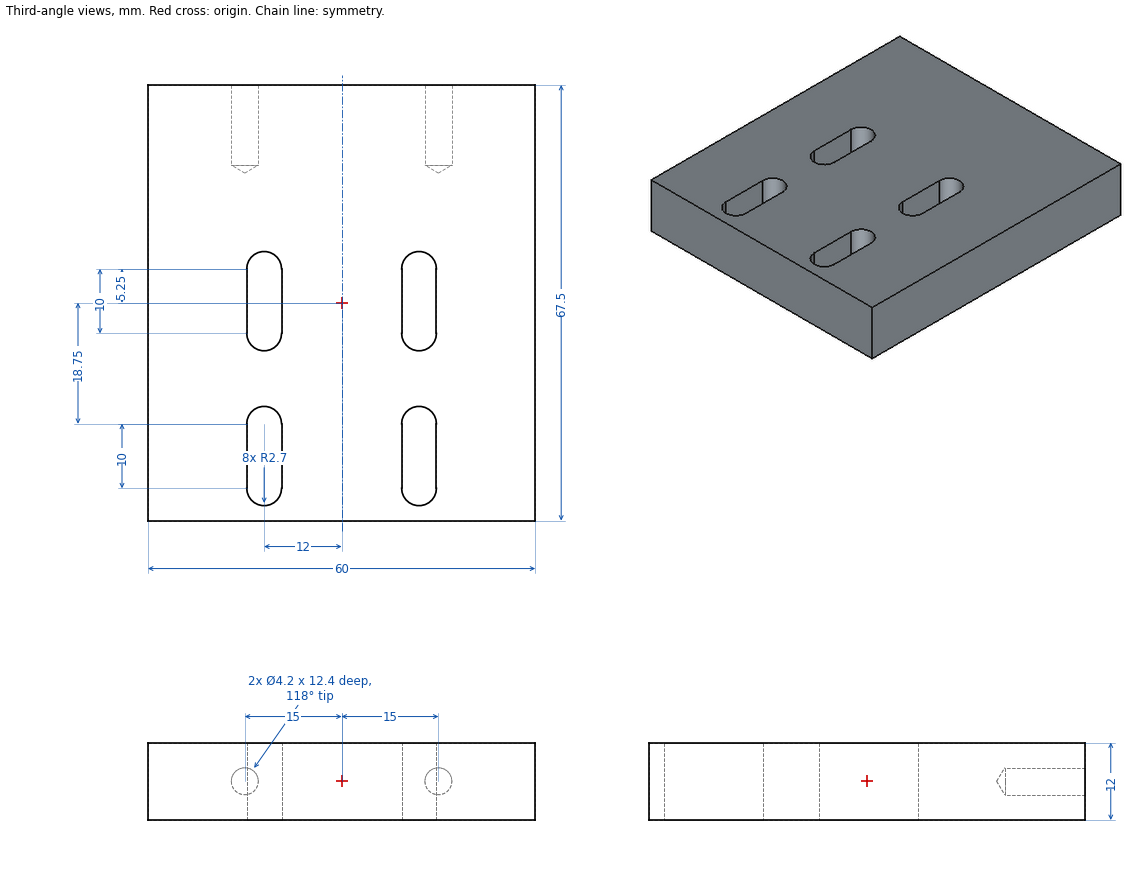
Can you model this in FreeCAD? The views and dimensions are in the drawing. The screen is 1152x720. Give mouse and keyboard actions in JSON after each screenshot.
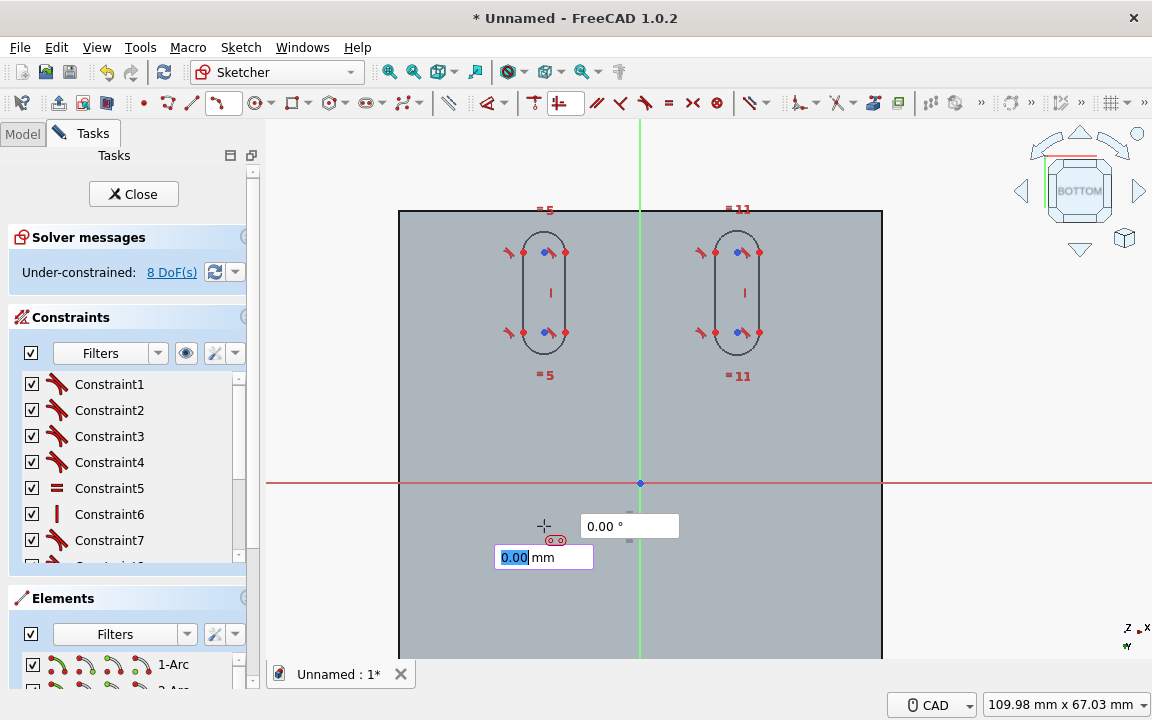
{"action": "left_click", "coordinate": [544, 445]}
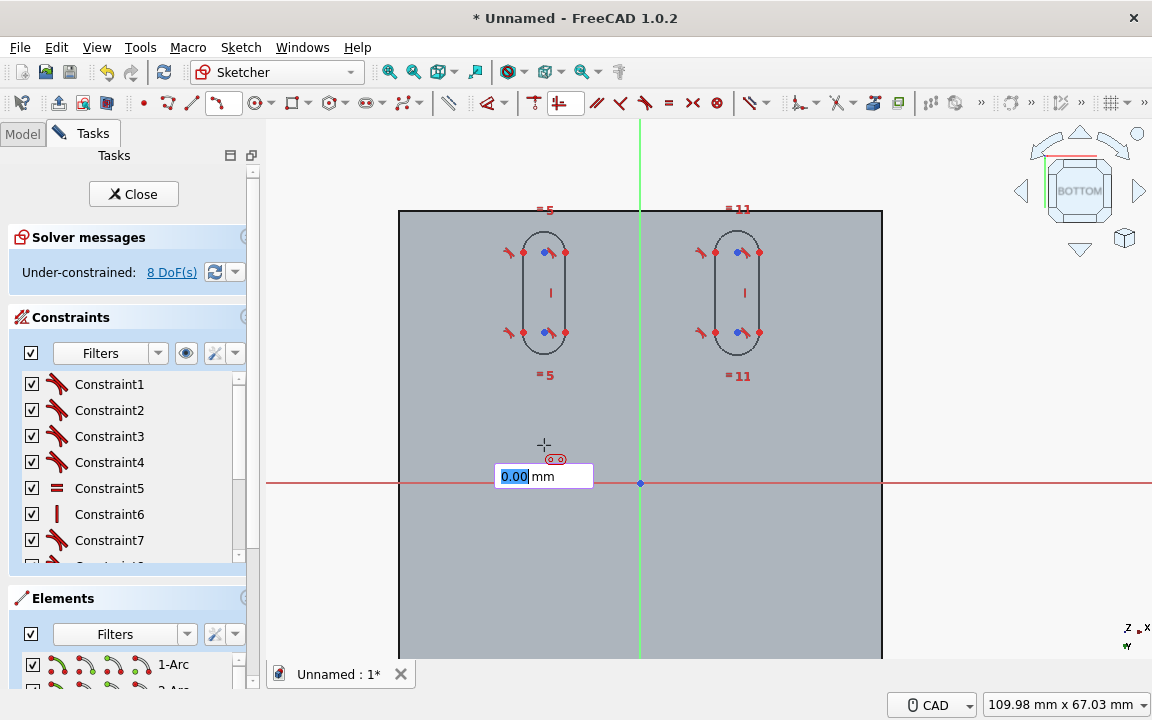
{"action": "left_click", "coordinate": [522, 497]}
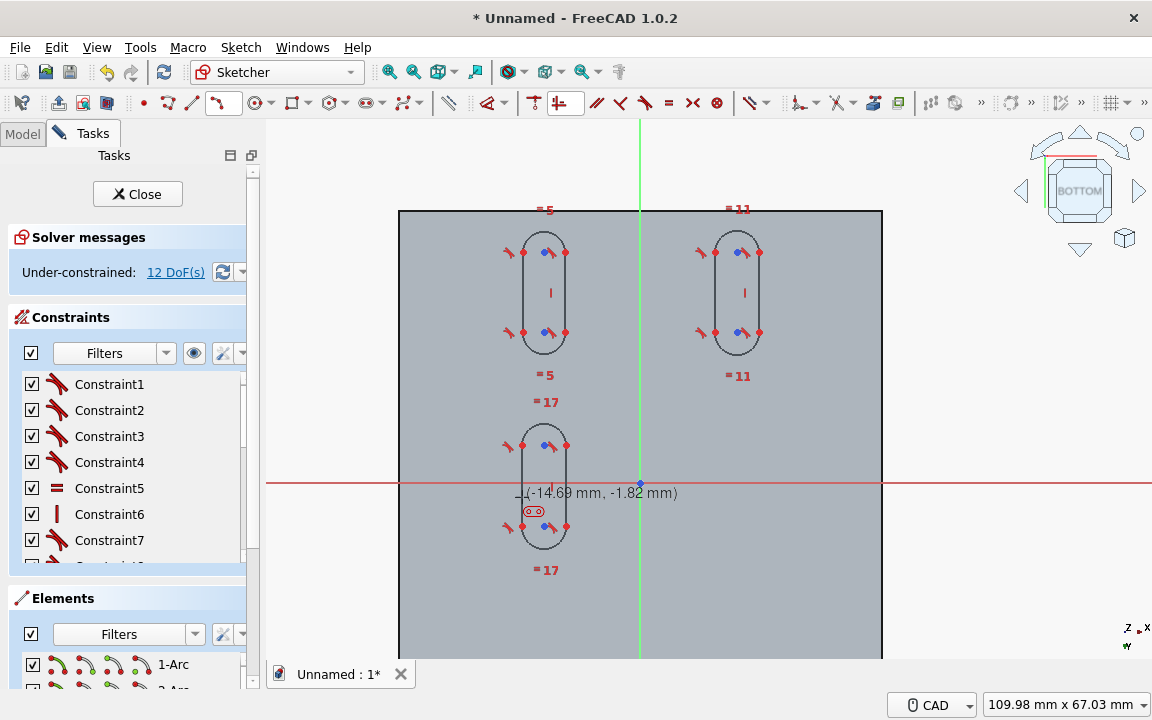
{"action": "left_click", "coordinate": [737, 526]}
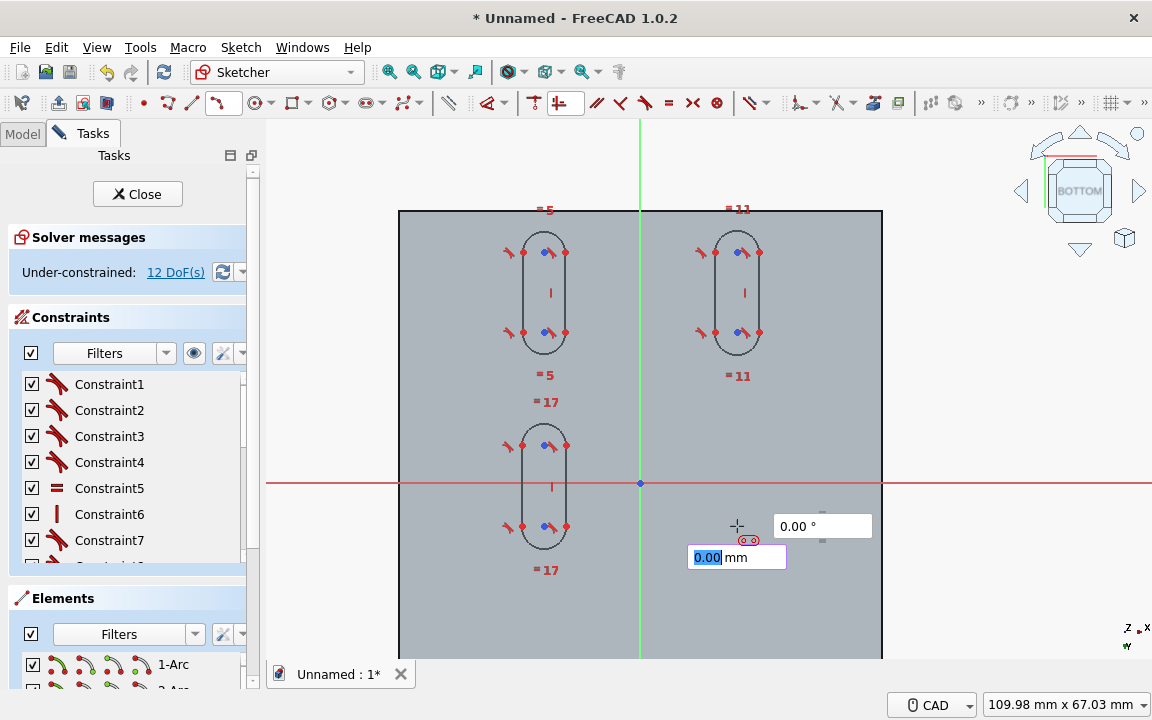
{"action": "left_click", "coordinate": [737, 445]}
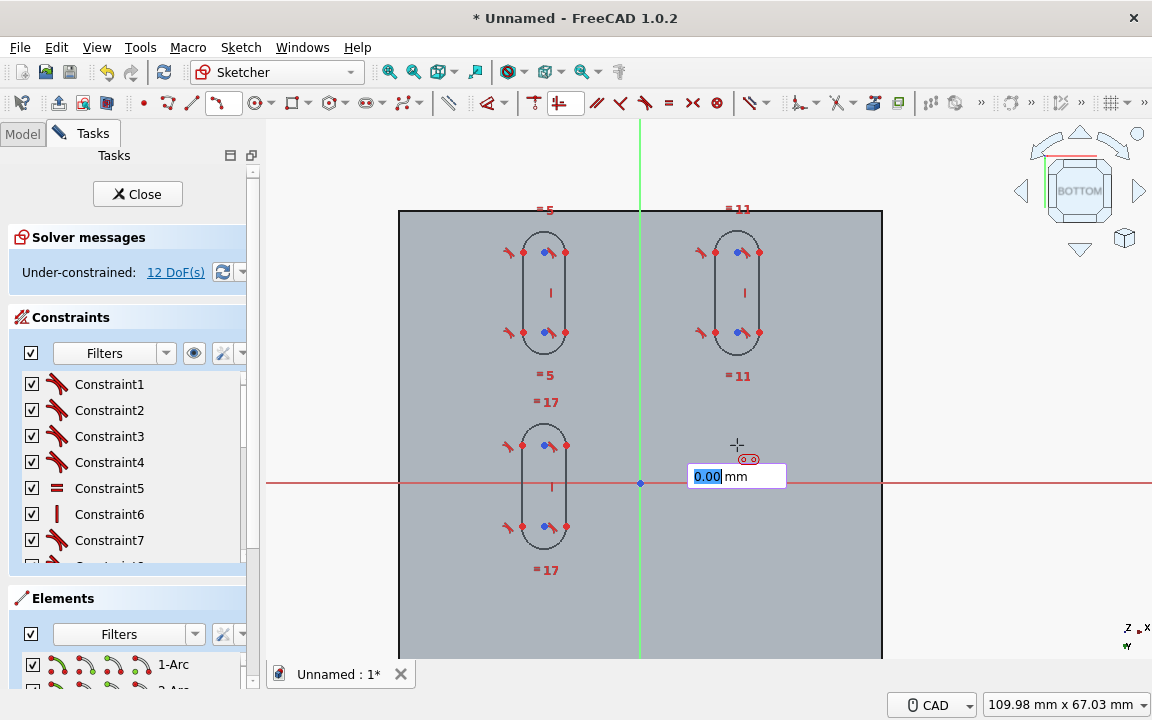
{"action": "left_click", "coordinate": [715, 497]}
{"action": "key", "text": "Escape"}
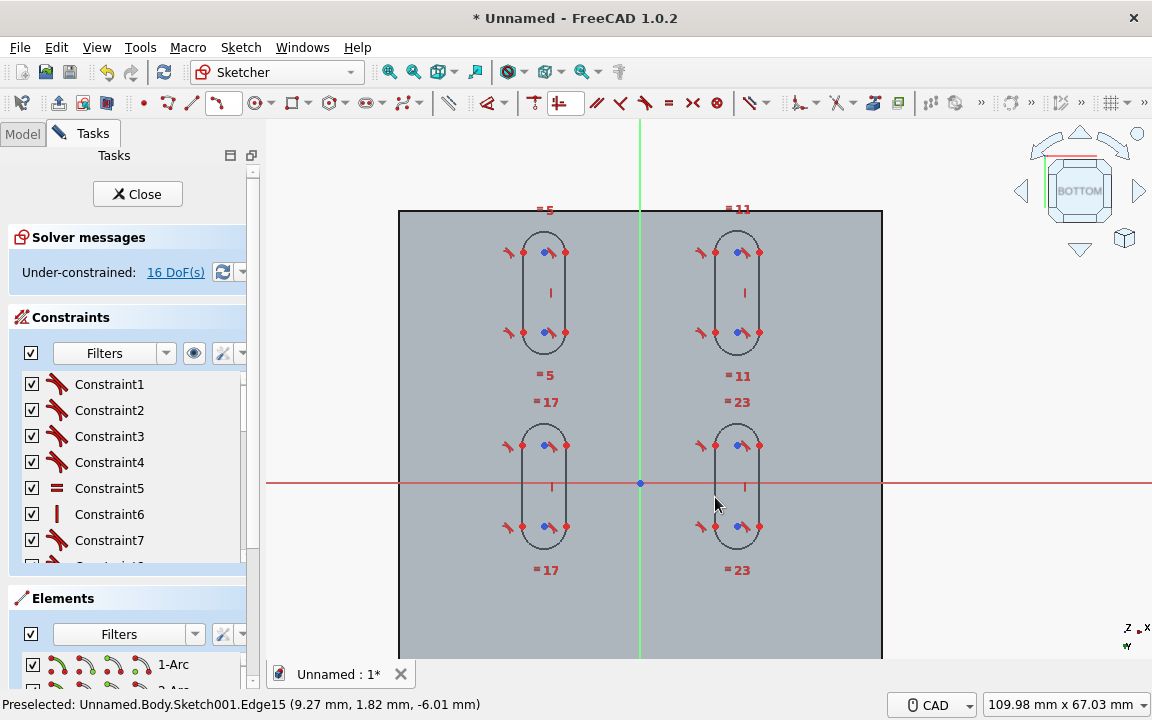
{"action": "left_click", "coordinate": [532, 350]}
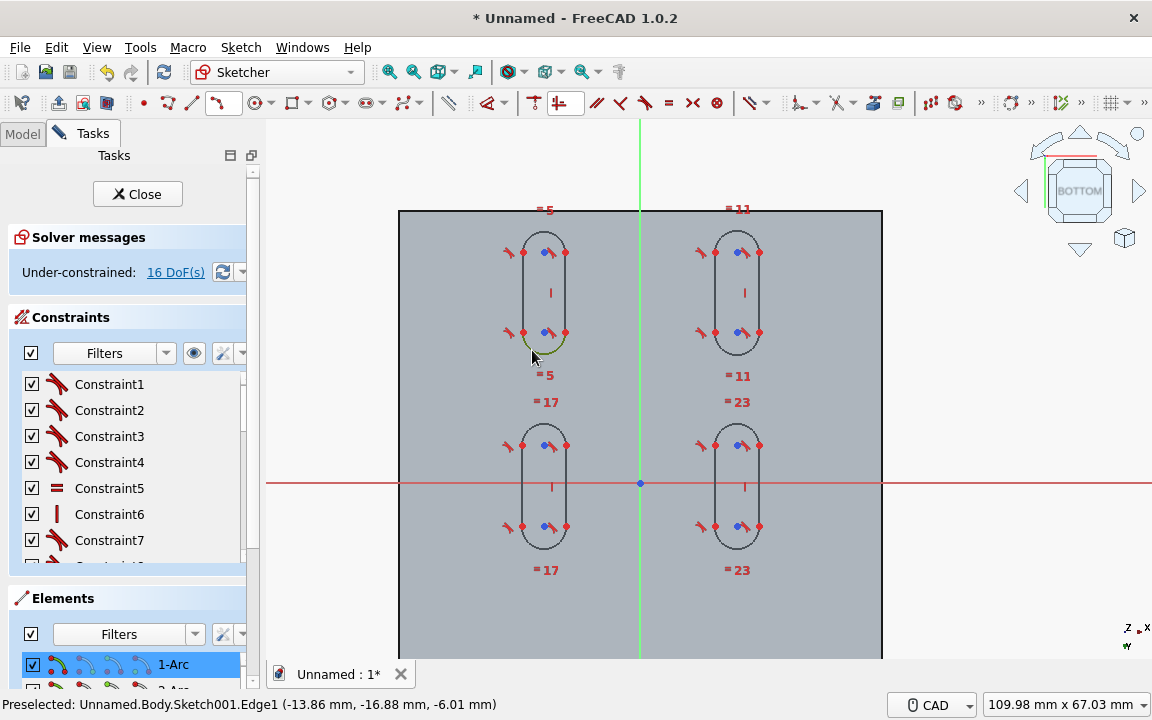
{"action": "left_click", "coordinate": [724, 351]}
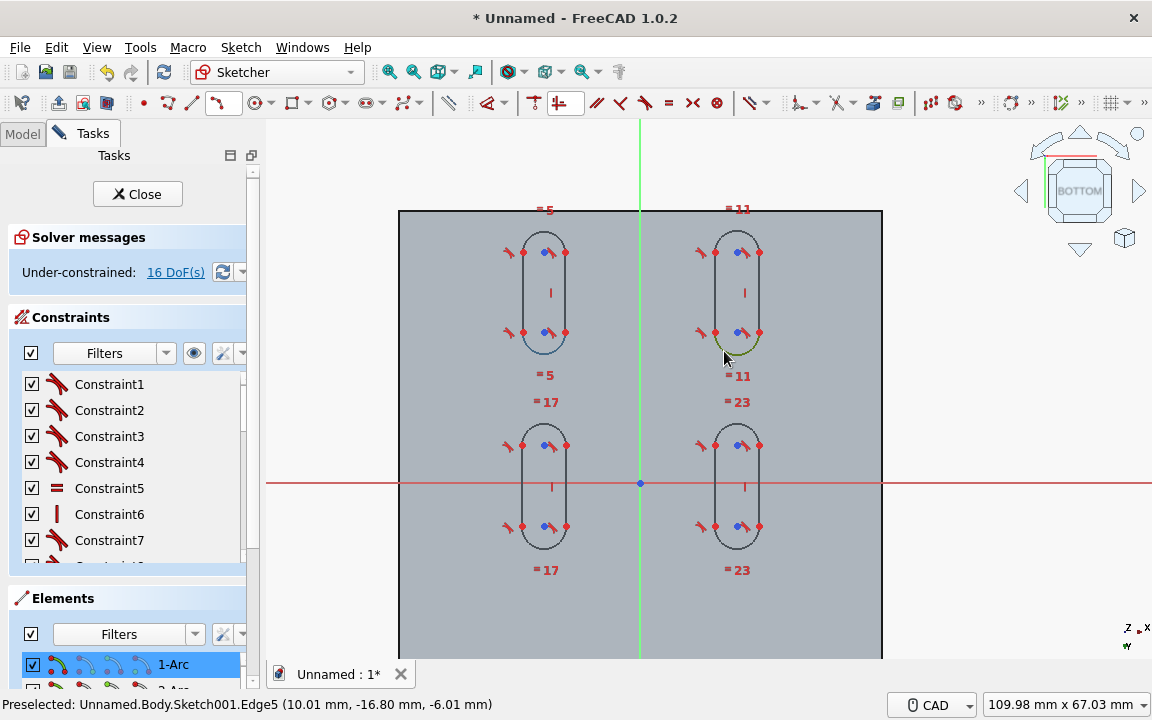
{"action": "left_click", "coordinate": [531, 545]}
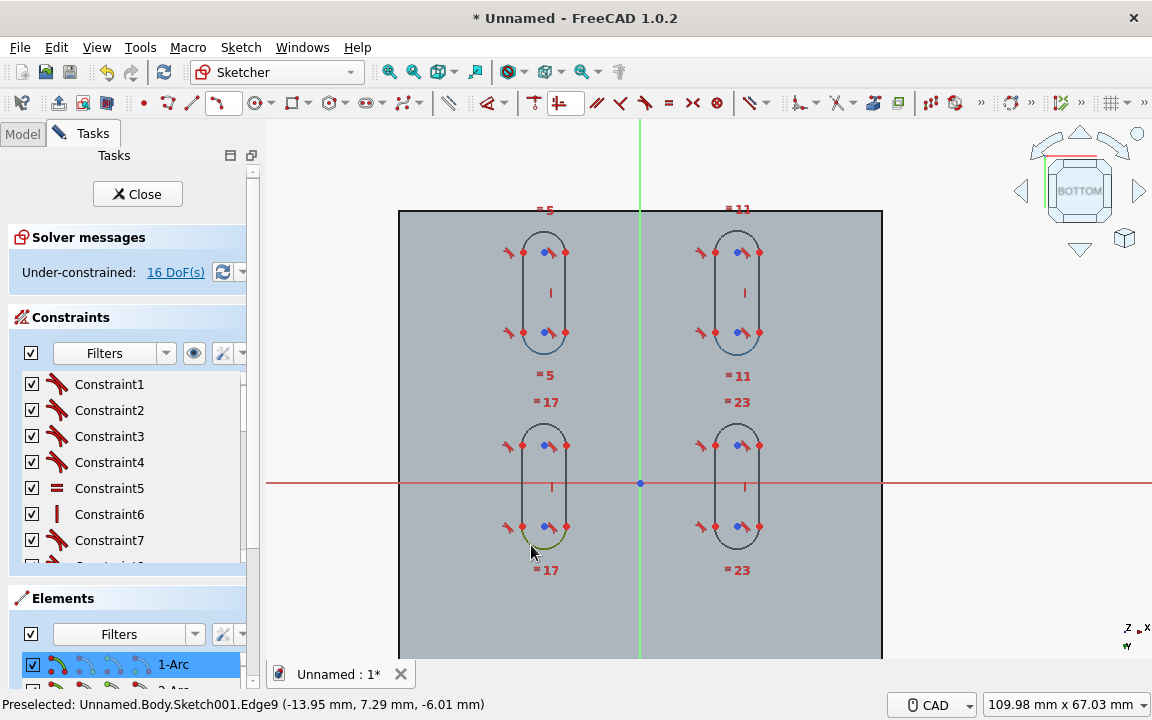
{"action": "left_click", "coordinate": [724, 545]}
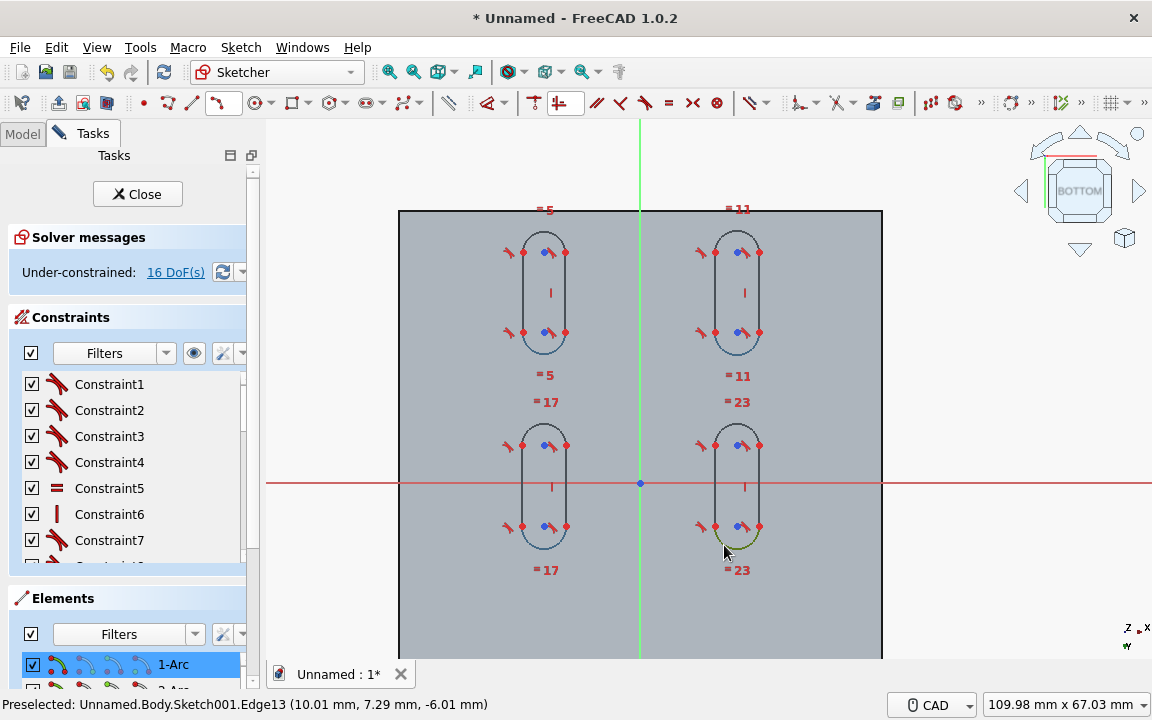
{"action": "key", "text": "e"}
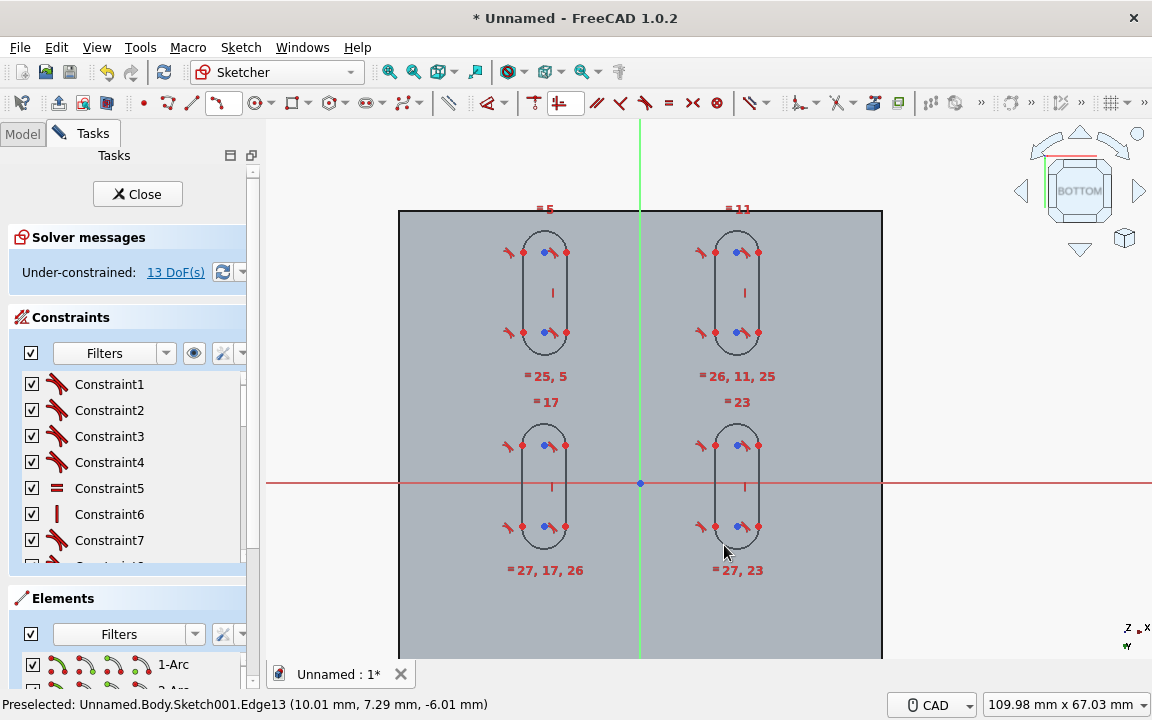
{"action": "left_click", "coordinate": [545, 333]}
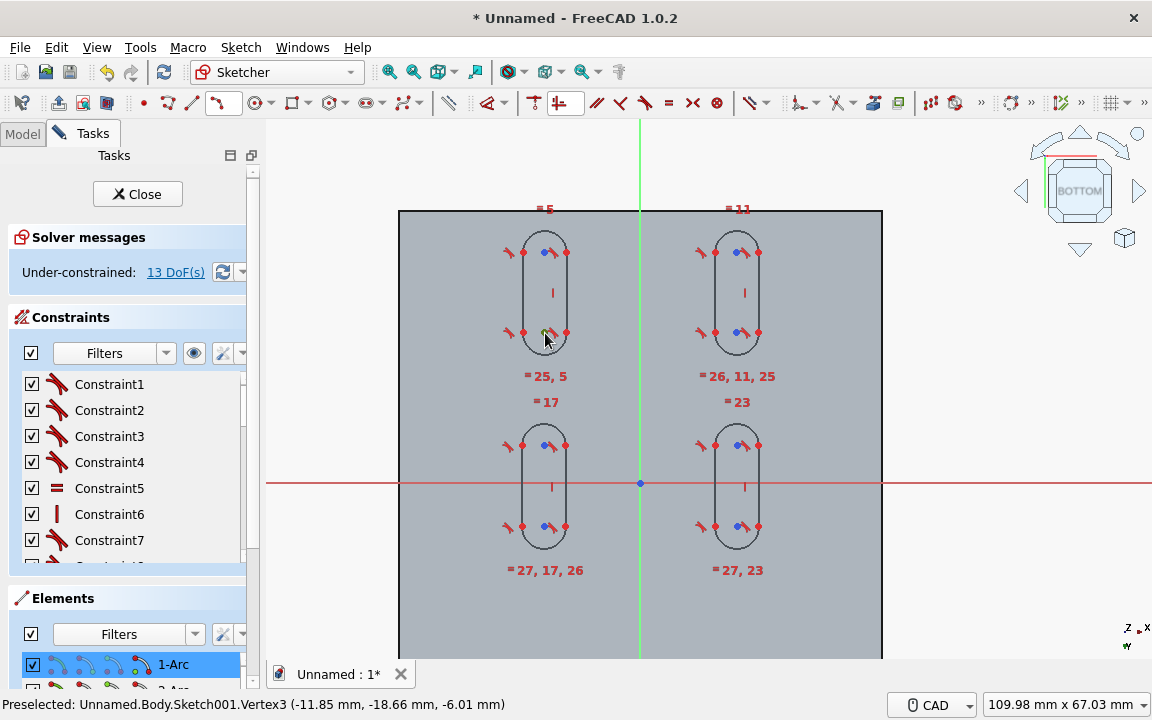
{"action": "left_click", "coordinate": [737, 333]}